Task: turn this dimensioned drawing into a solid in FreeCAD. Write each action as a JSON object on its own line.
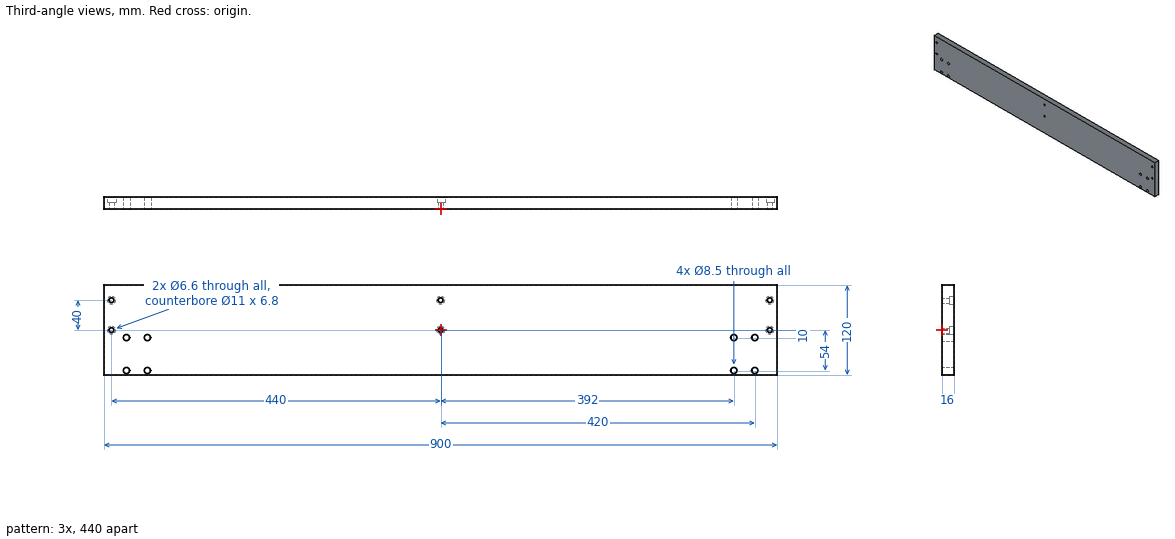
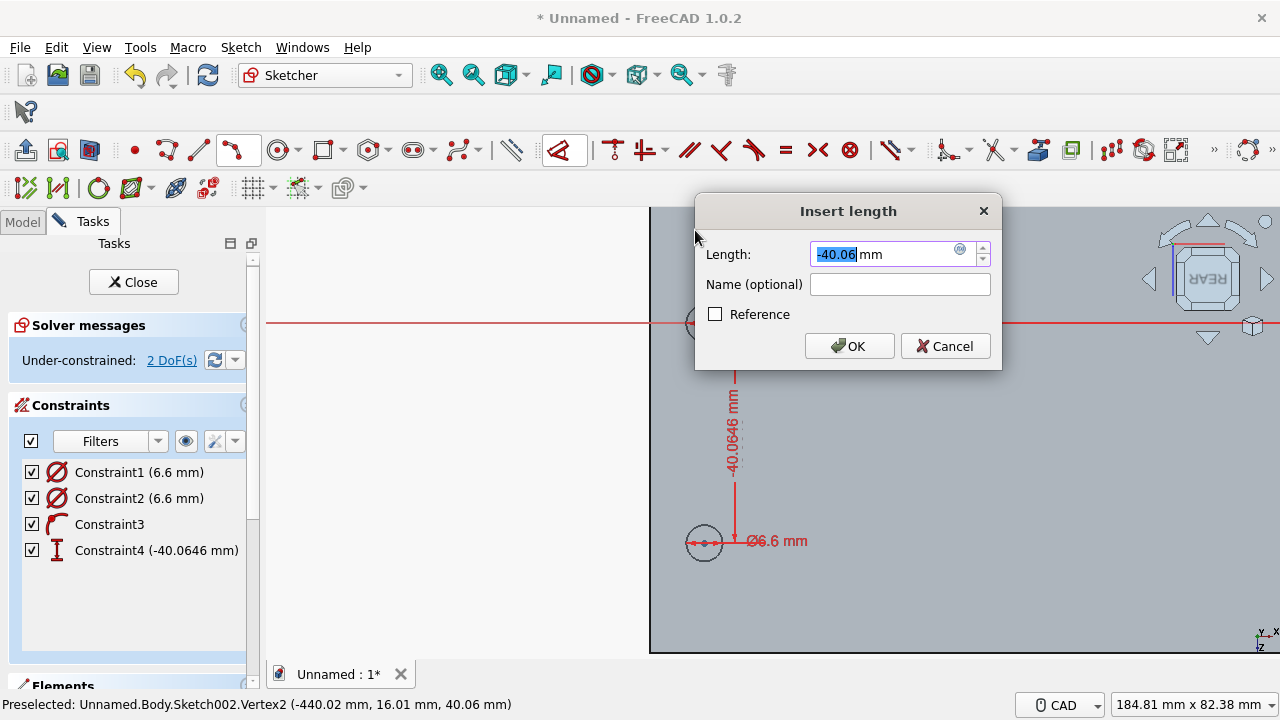
{"action": "type", "text": "-40"}
{"action": "key", "text": "Return"}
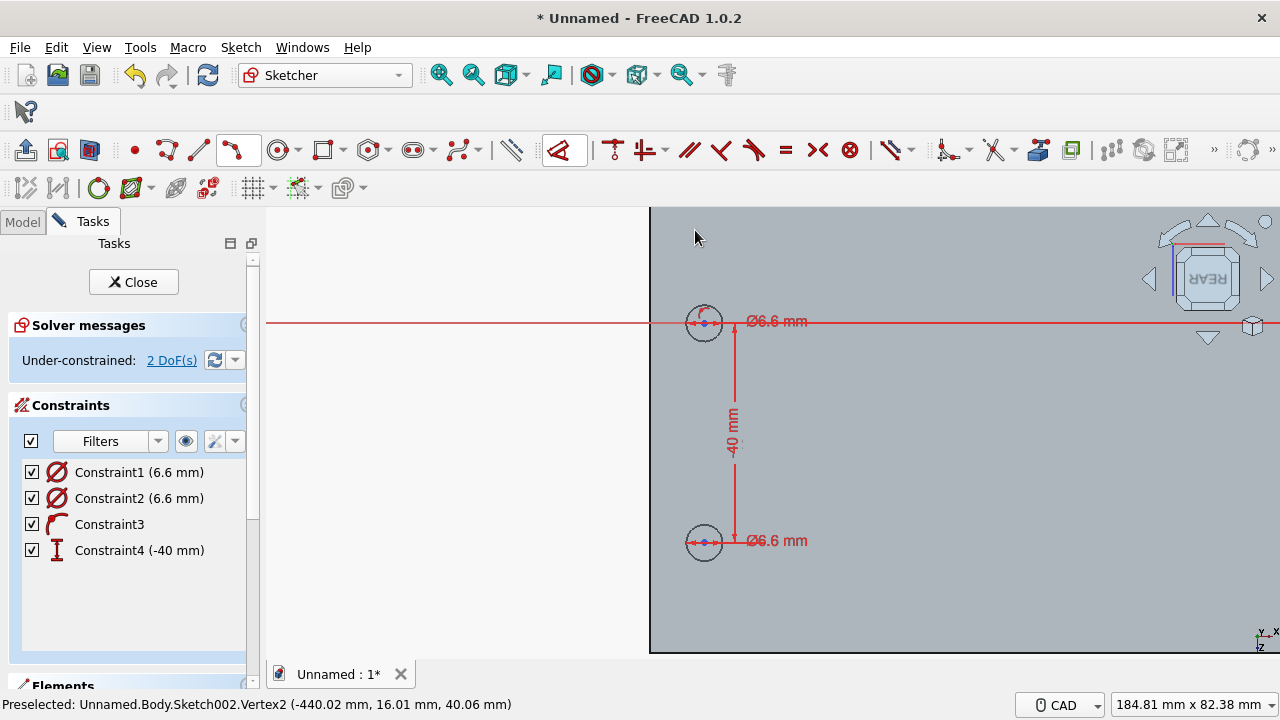
{"action": "left_click", "coordinate": [704, 323]}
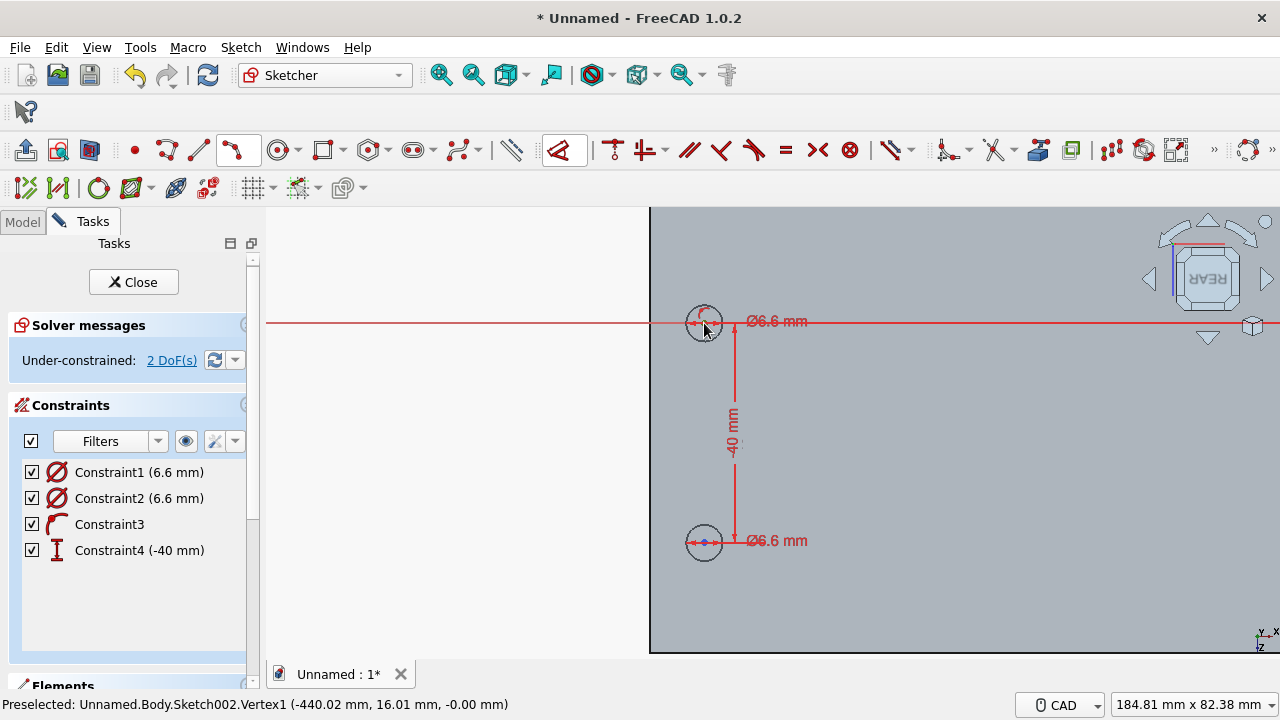
{"action": "key", "text": "l"}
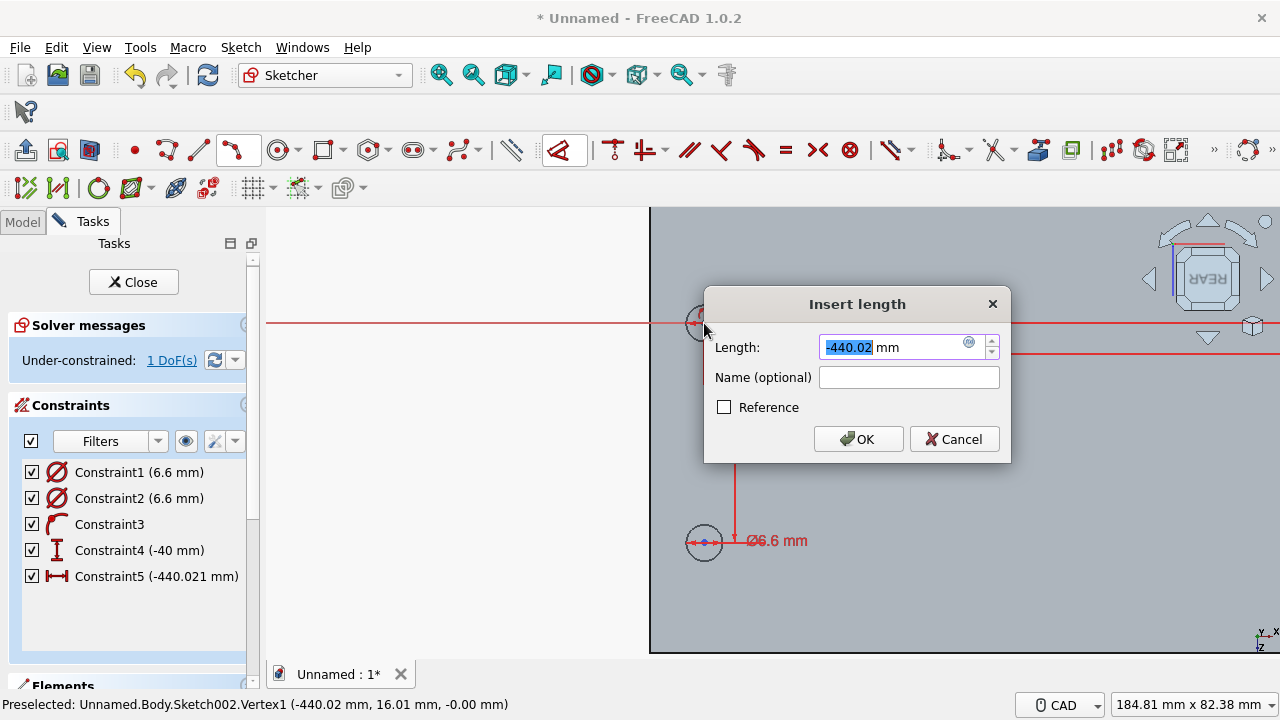
{"action": "type", "text": "-440"}
{"action": "key", "text": "Return"}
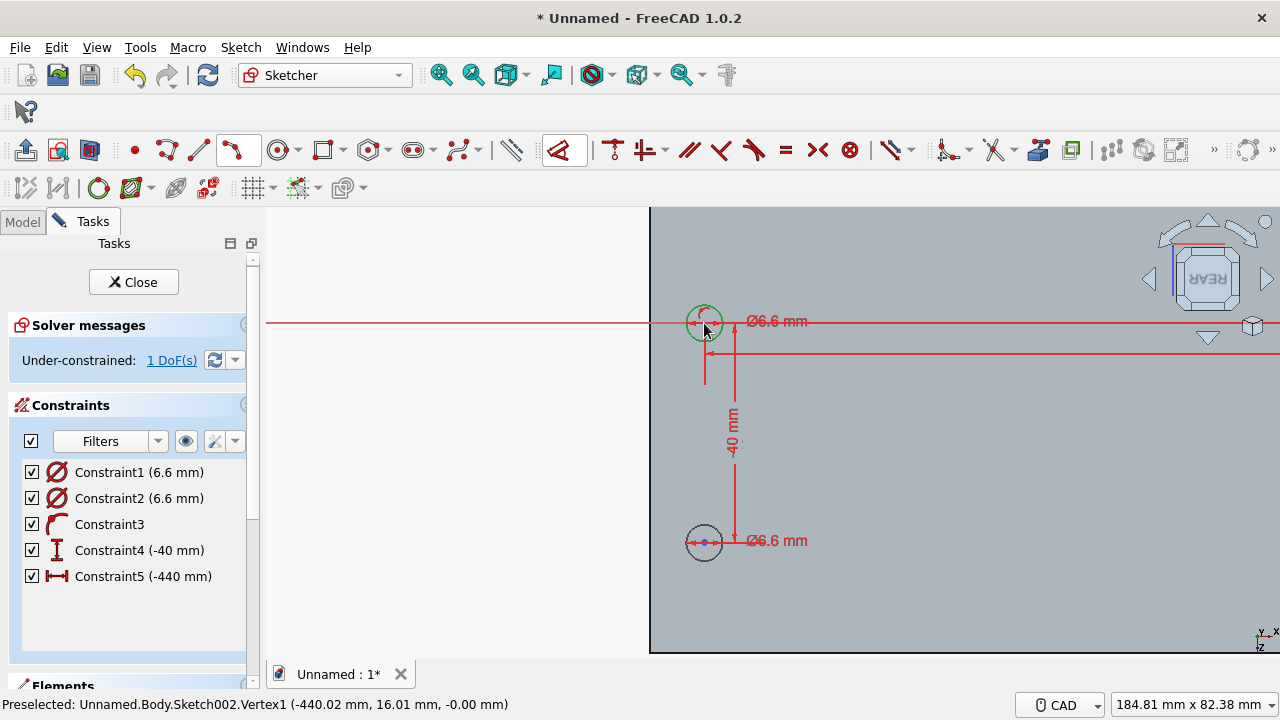
{"action": "left_click", "coordinate": [704, 543]}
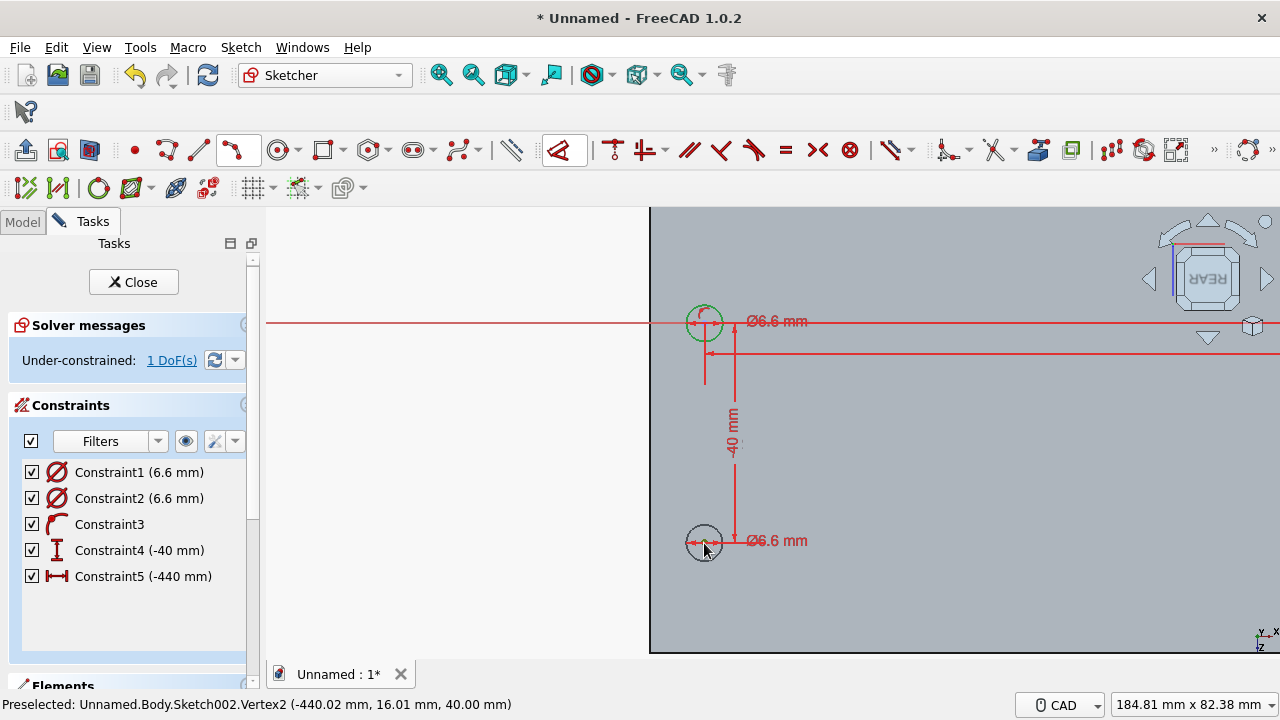
{"action": "key", "text": "l"}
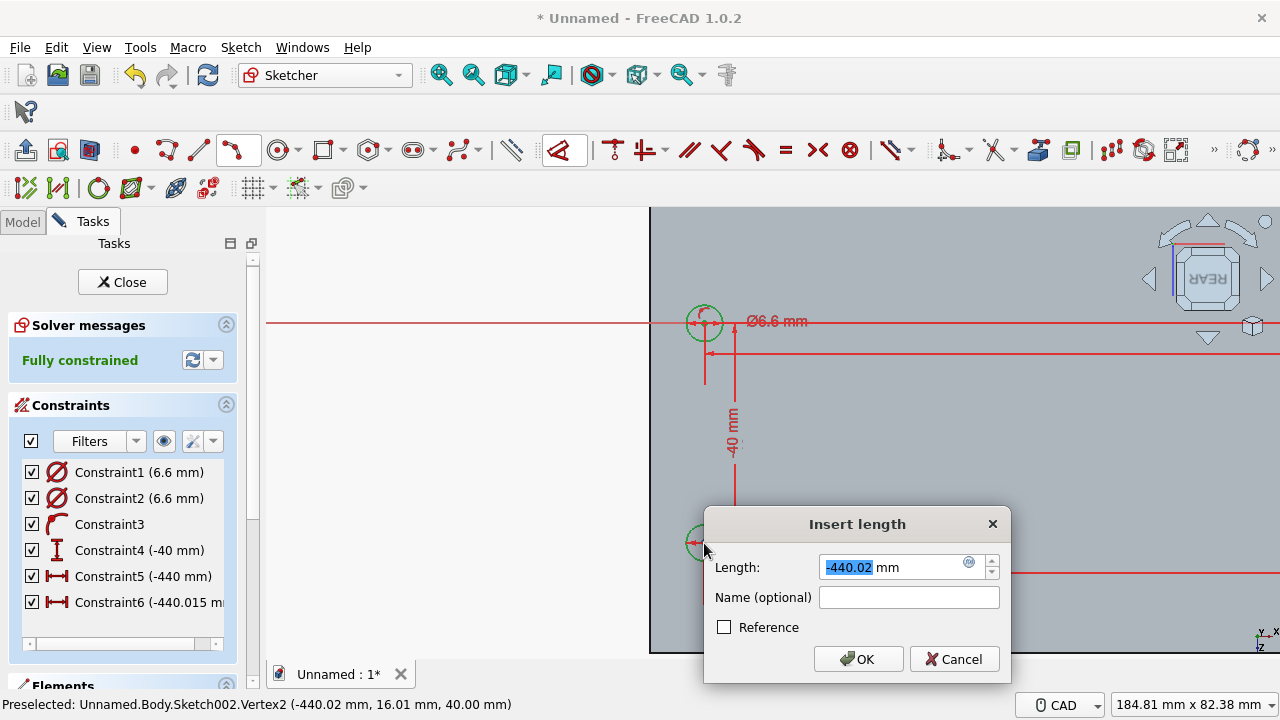
{"action": "type", "text": "-440"}
{"action": "key", "text": "Return"}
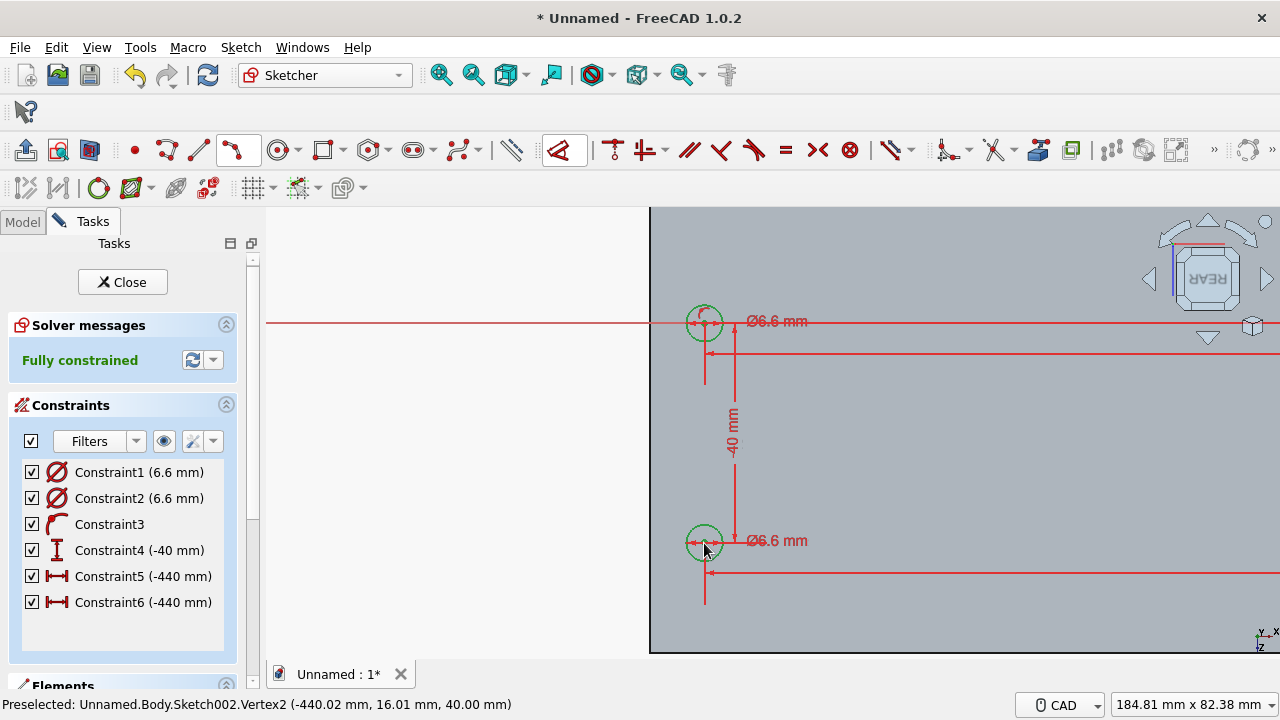
{"action": "left_click", "coordinate": [123, 282]}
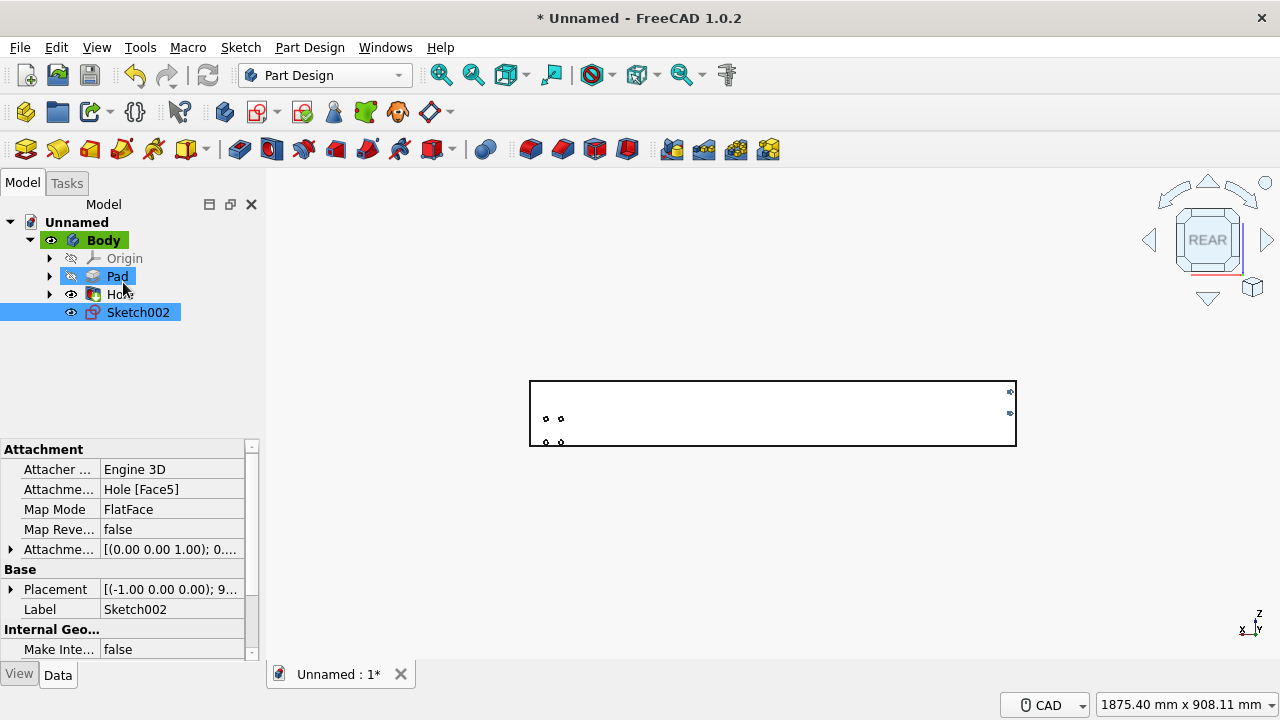
{"action": "left_click", "coordinate": [272, 150]}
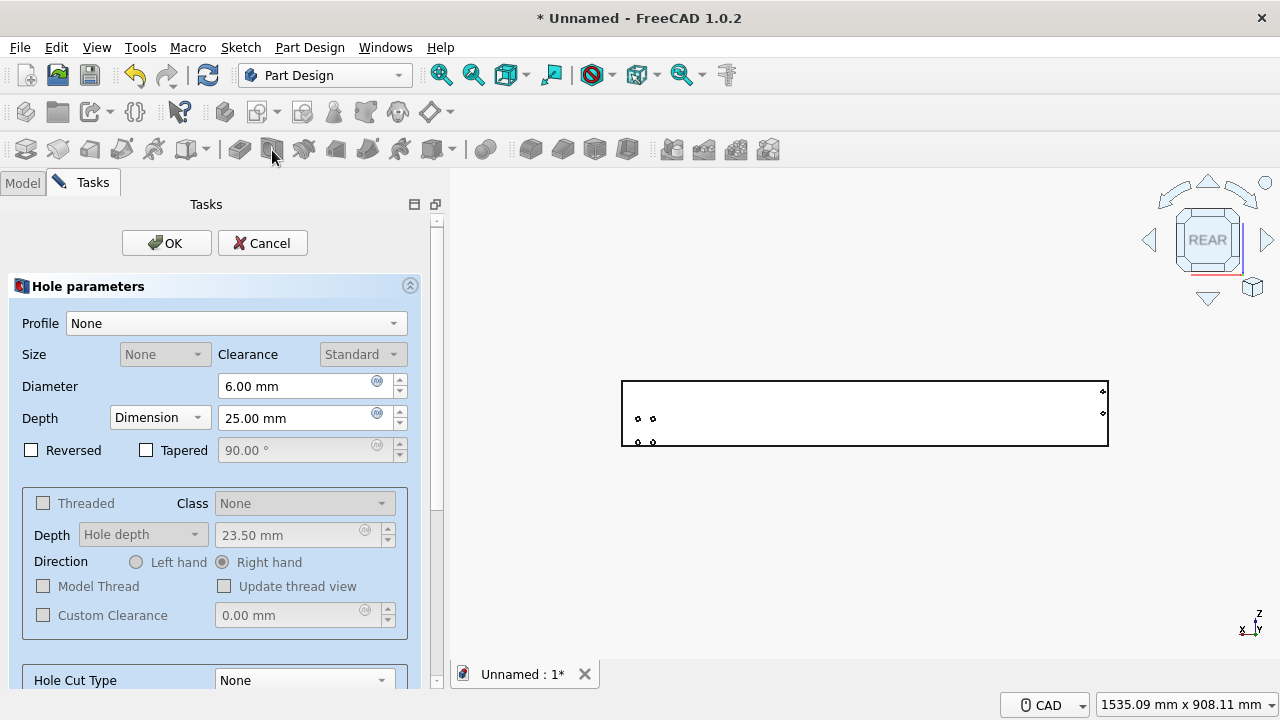
{"action": "triple_click", "coordinate": [305, 386]}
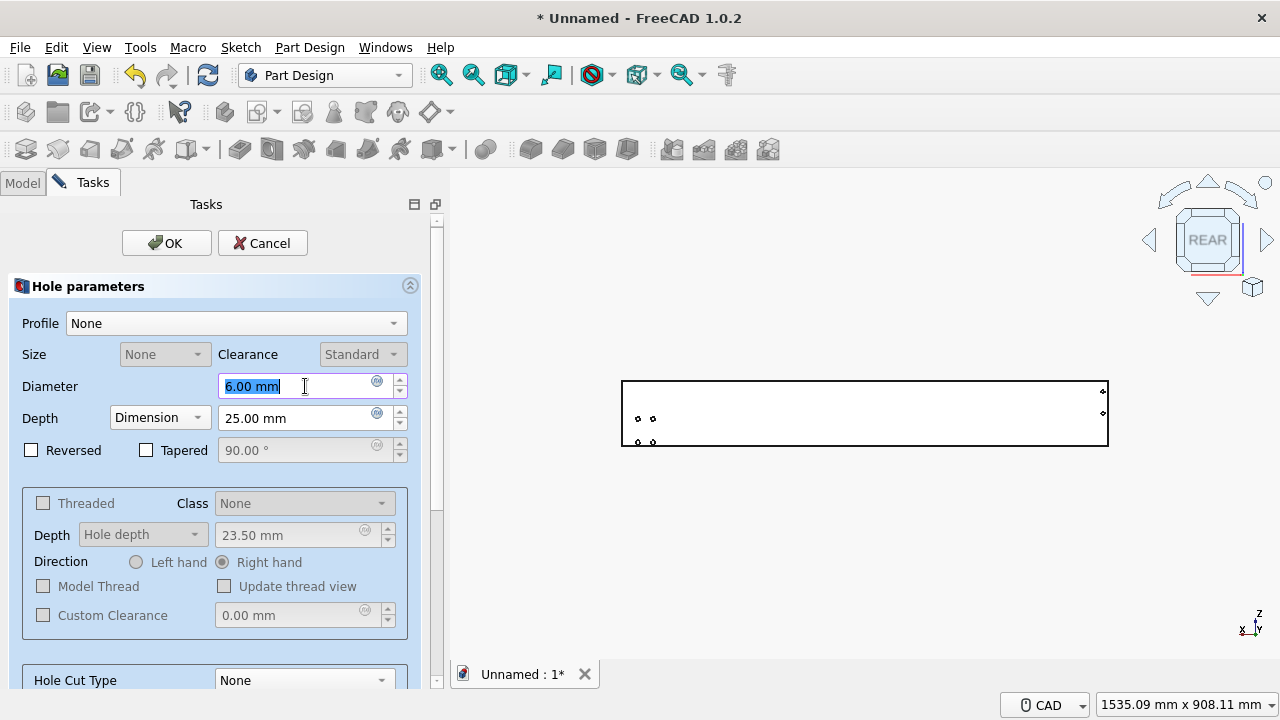
{"action": "type", "text": "6.6"}
{"action": "key", "text": "Tab"}